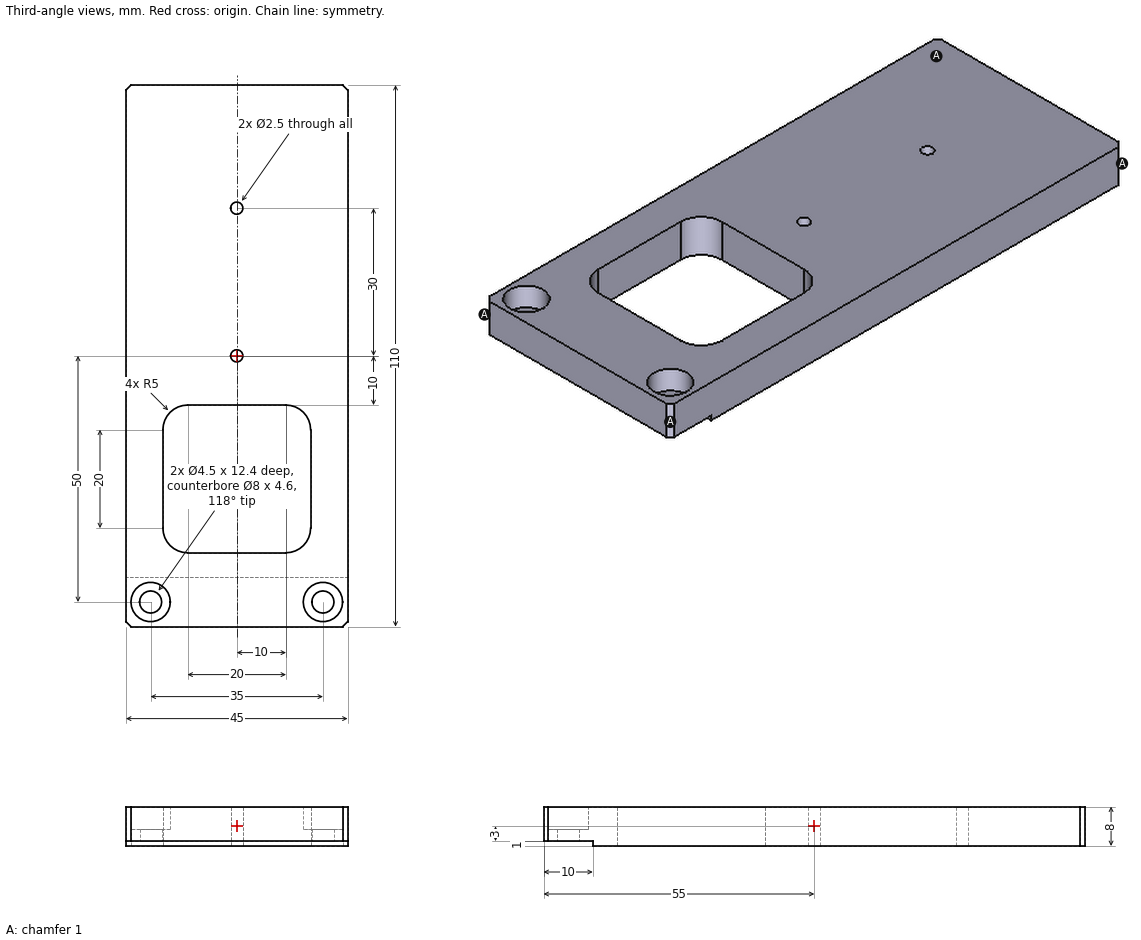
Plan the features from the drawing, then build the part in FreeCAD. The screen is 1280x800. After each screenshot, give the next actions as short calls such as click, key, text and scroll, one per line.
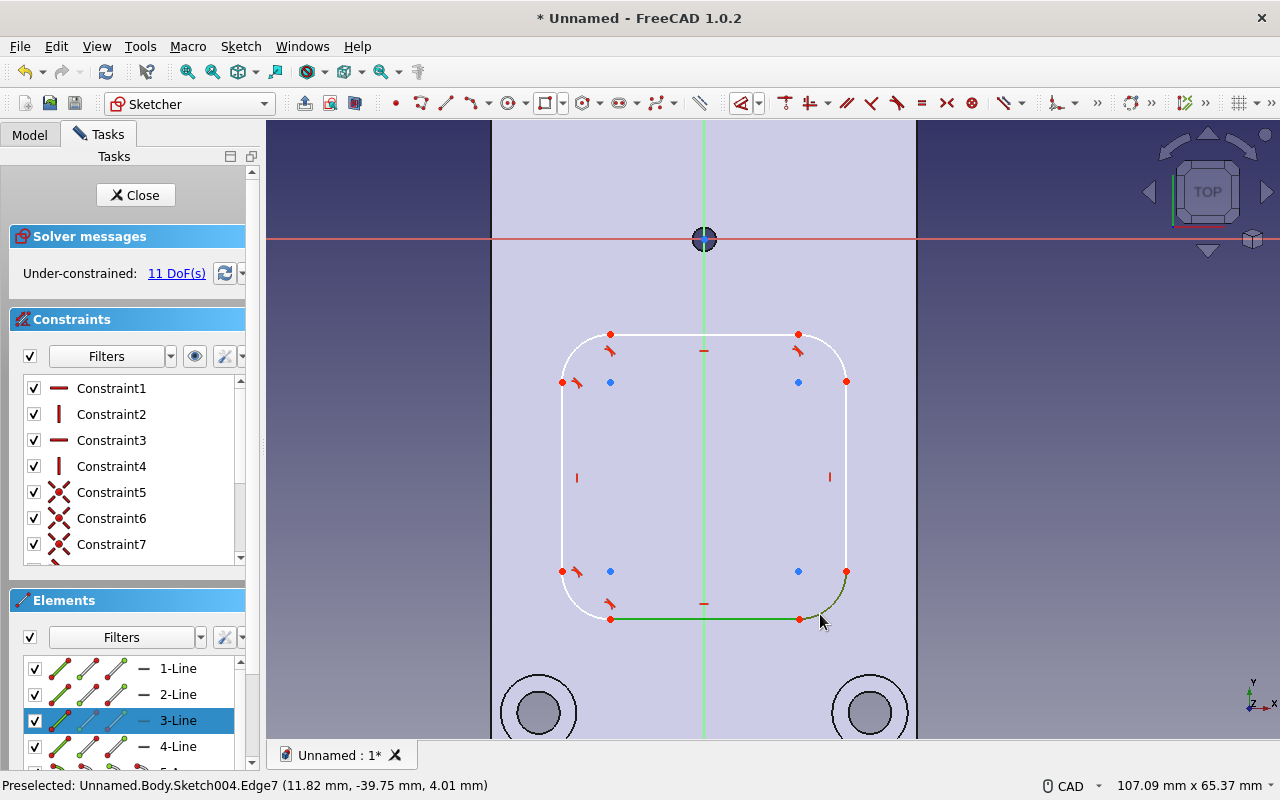
click(897, 104)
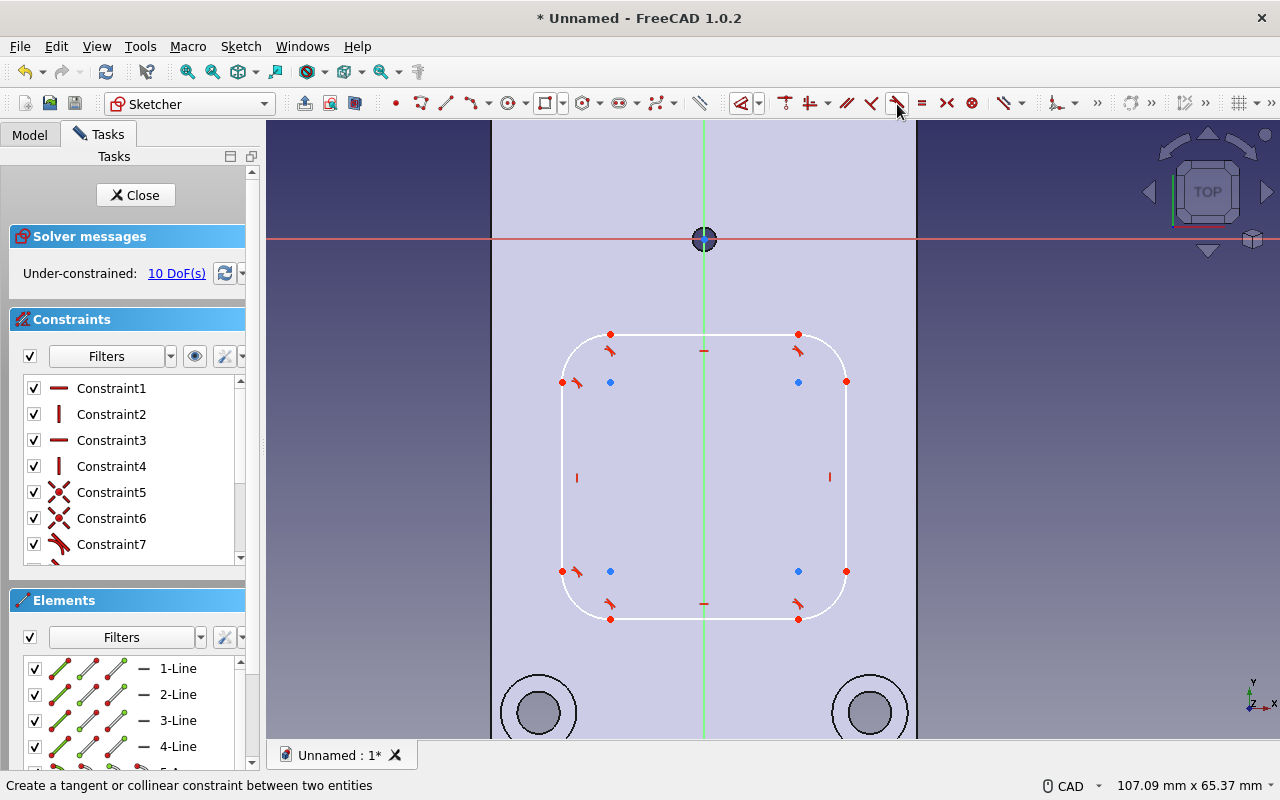
click(846, 515)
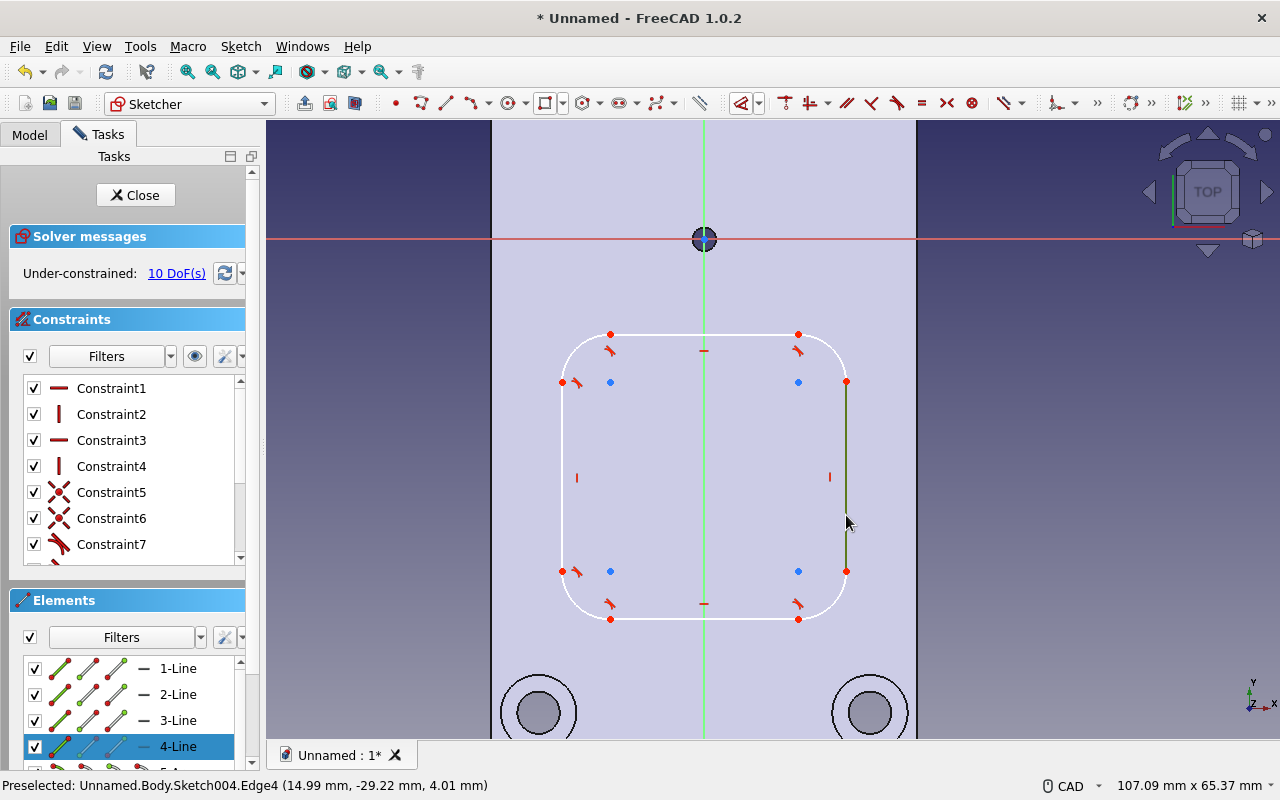
click(820, 614)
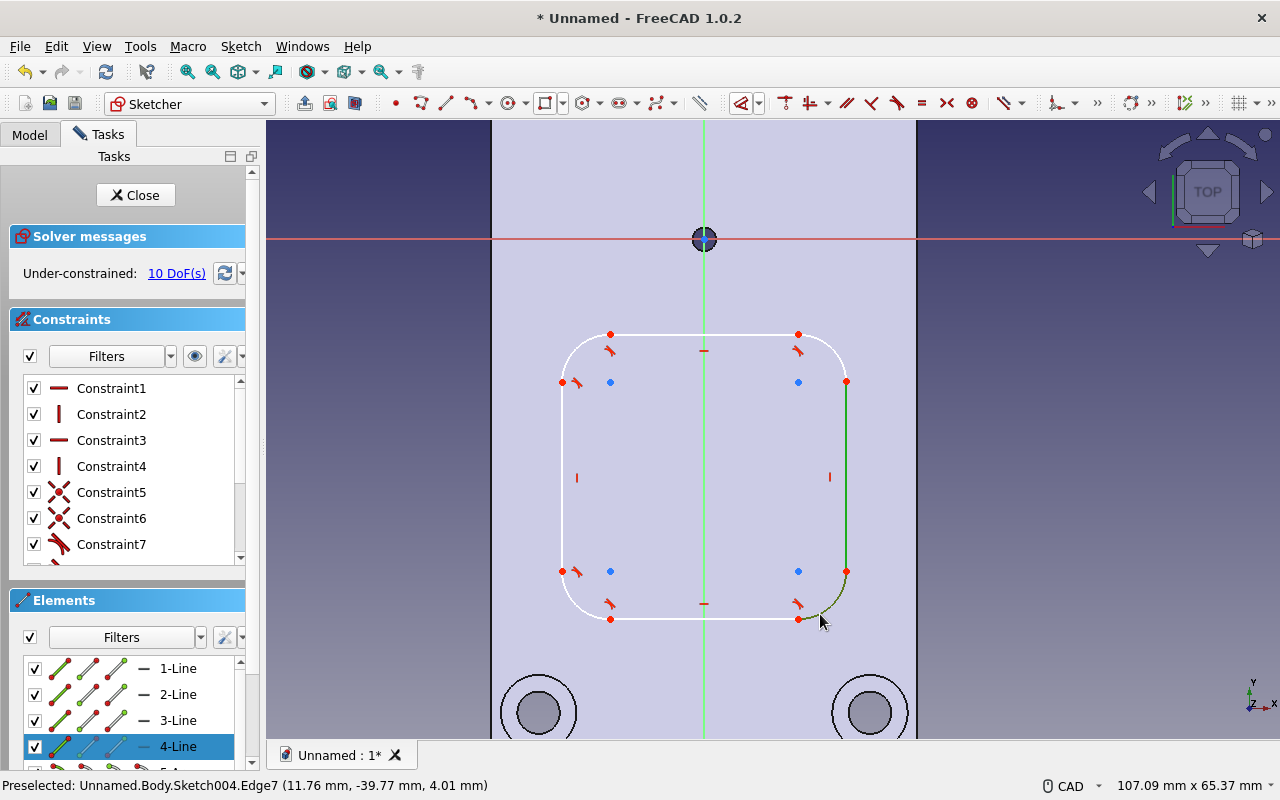
click(897, 104)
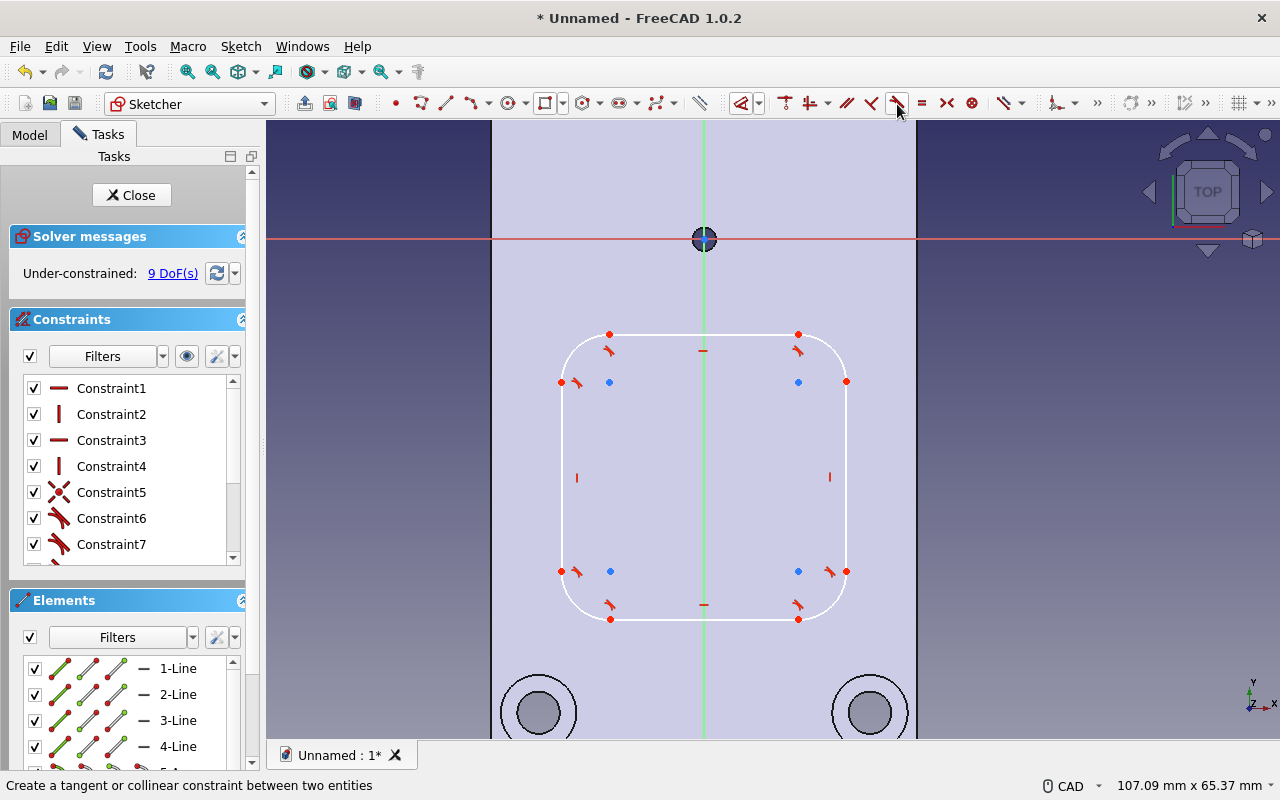
click(846, 515)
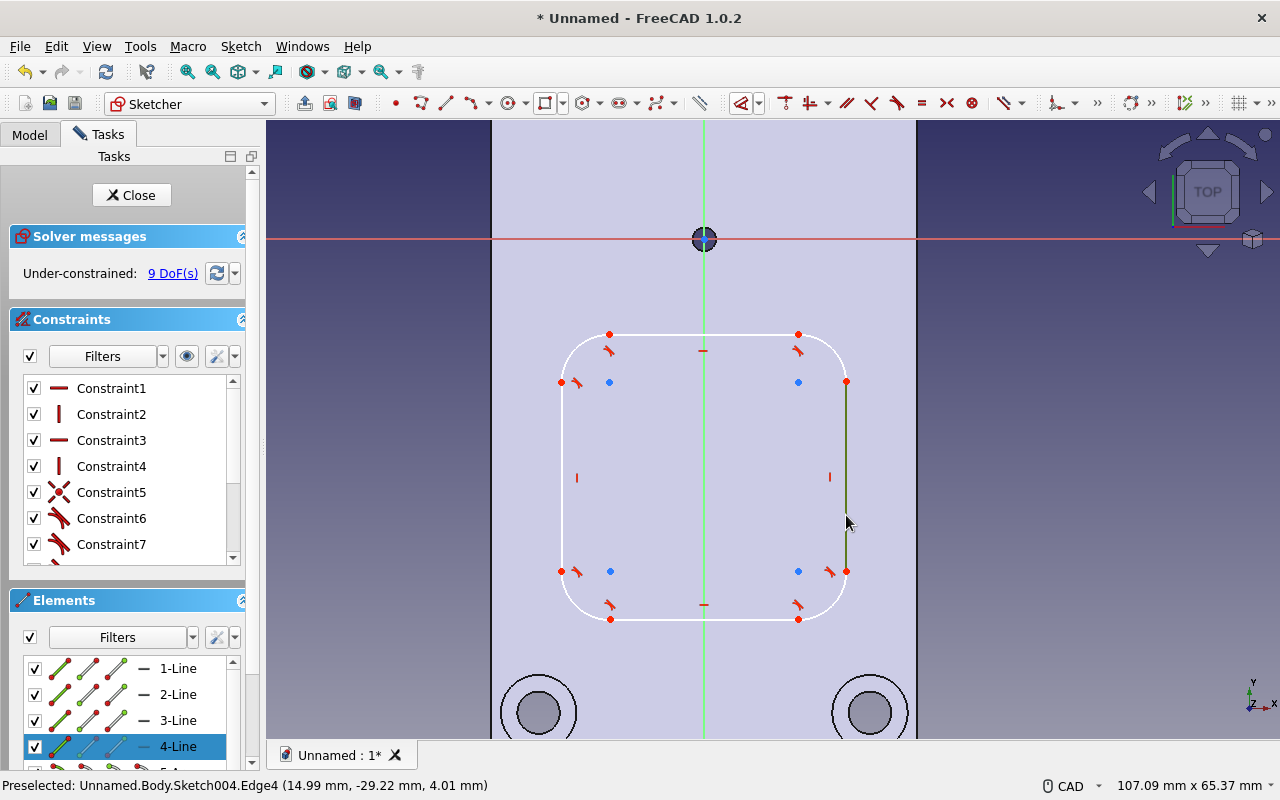
click(841, 361)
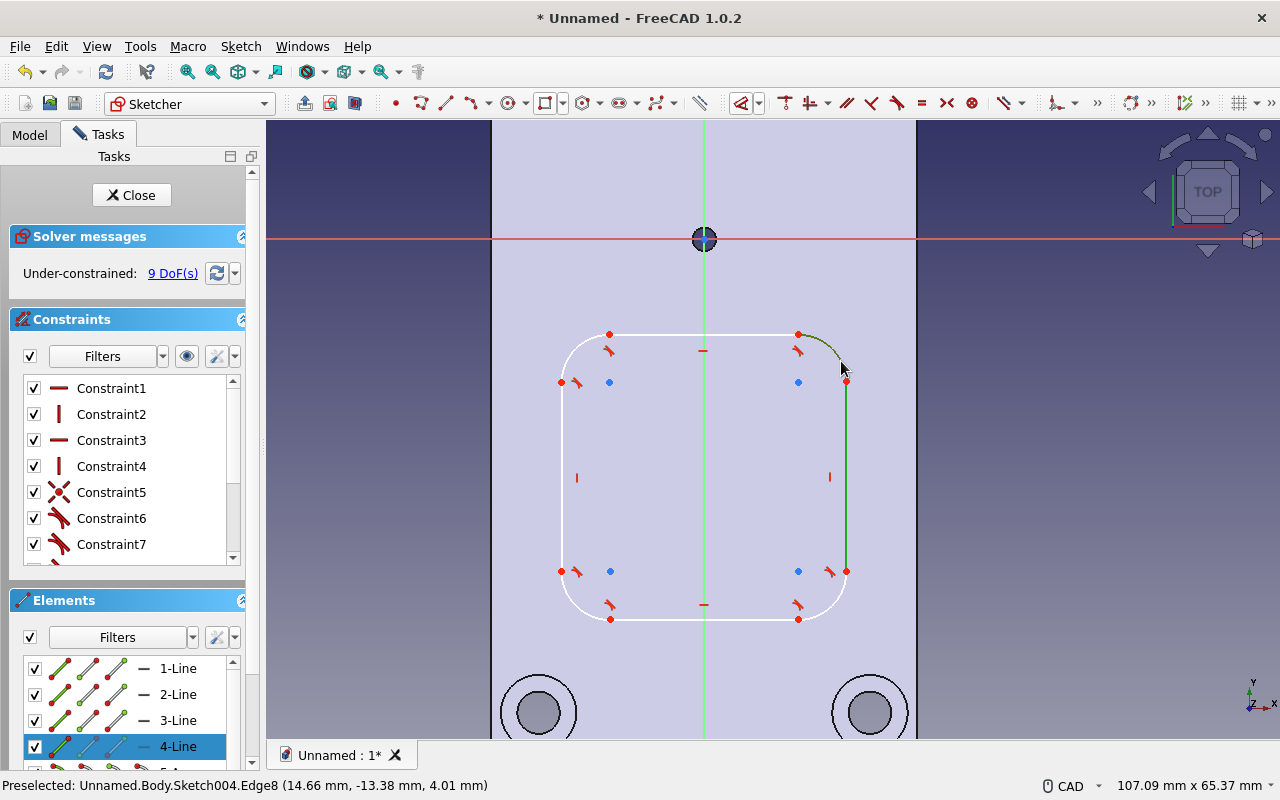
click(897, 104)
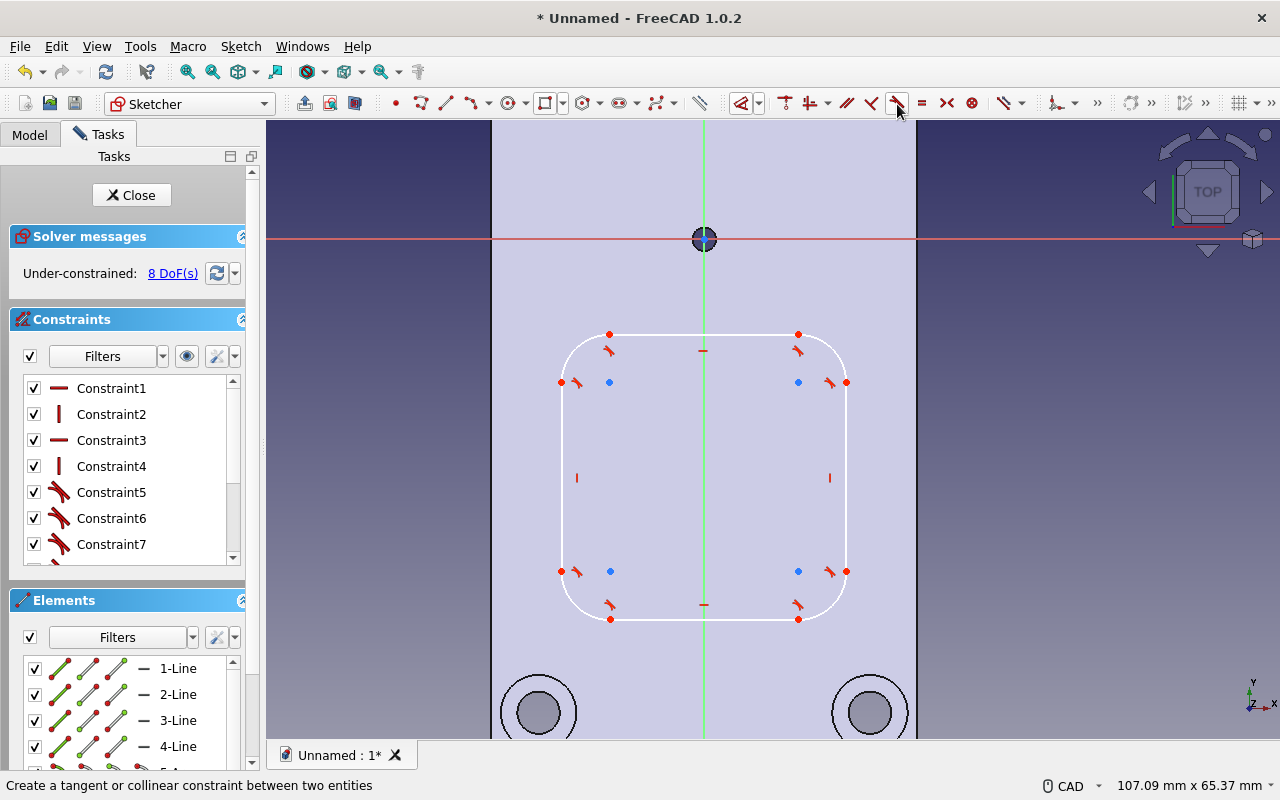
click(588, 340)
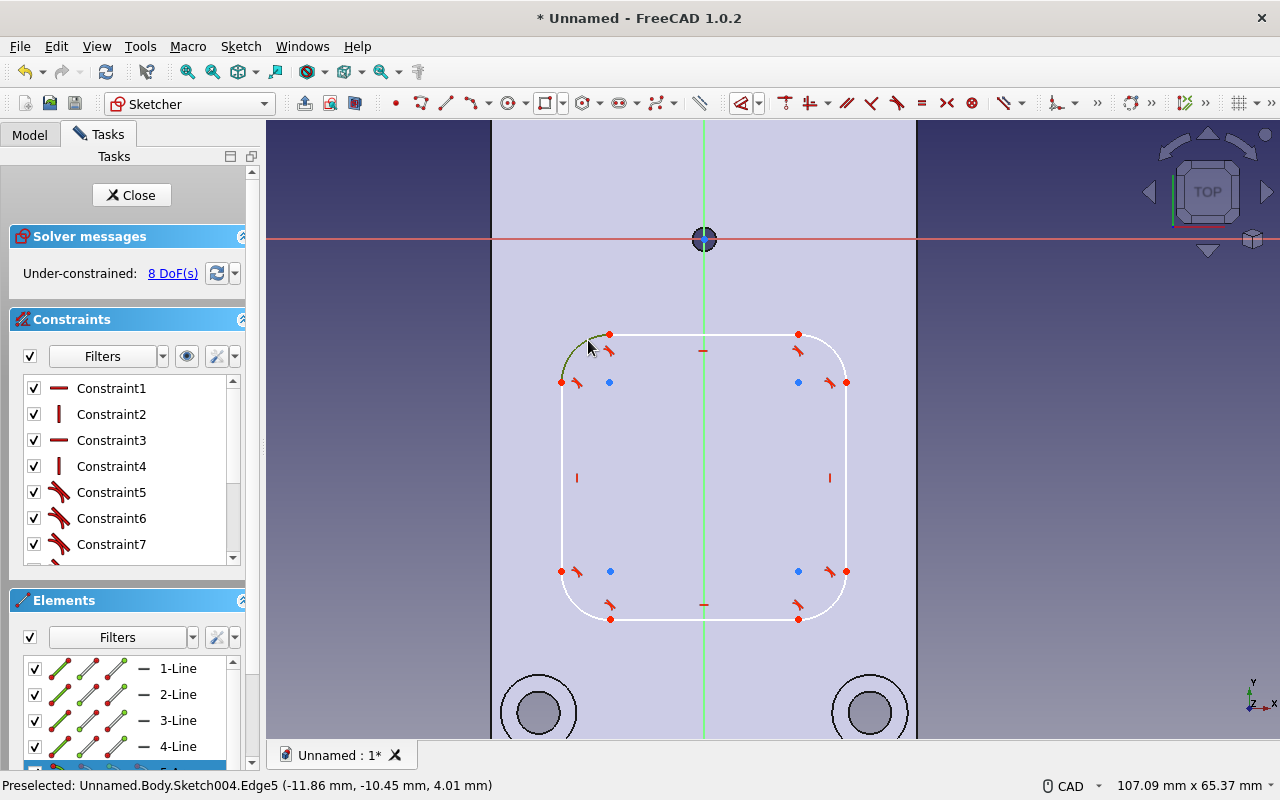
click(567, 594)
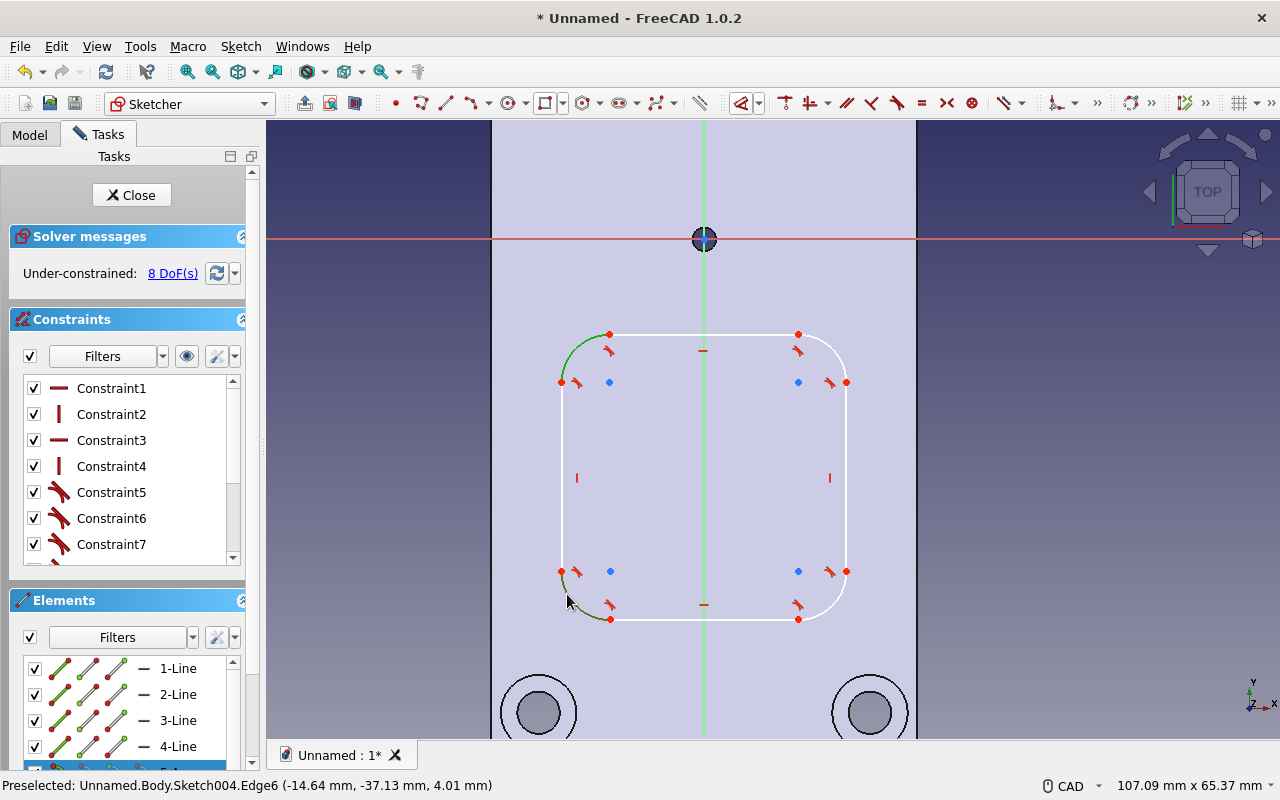
click(820, 615)